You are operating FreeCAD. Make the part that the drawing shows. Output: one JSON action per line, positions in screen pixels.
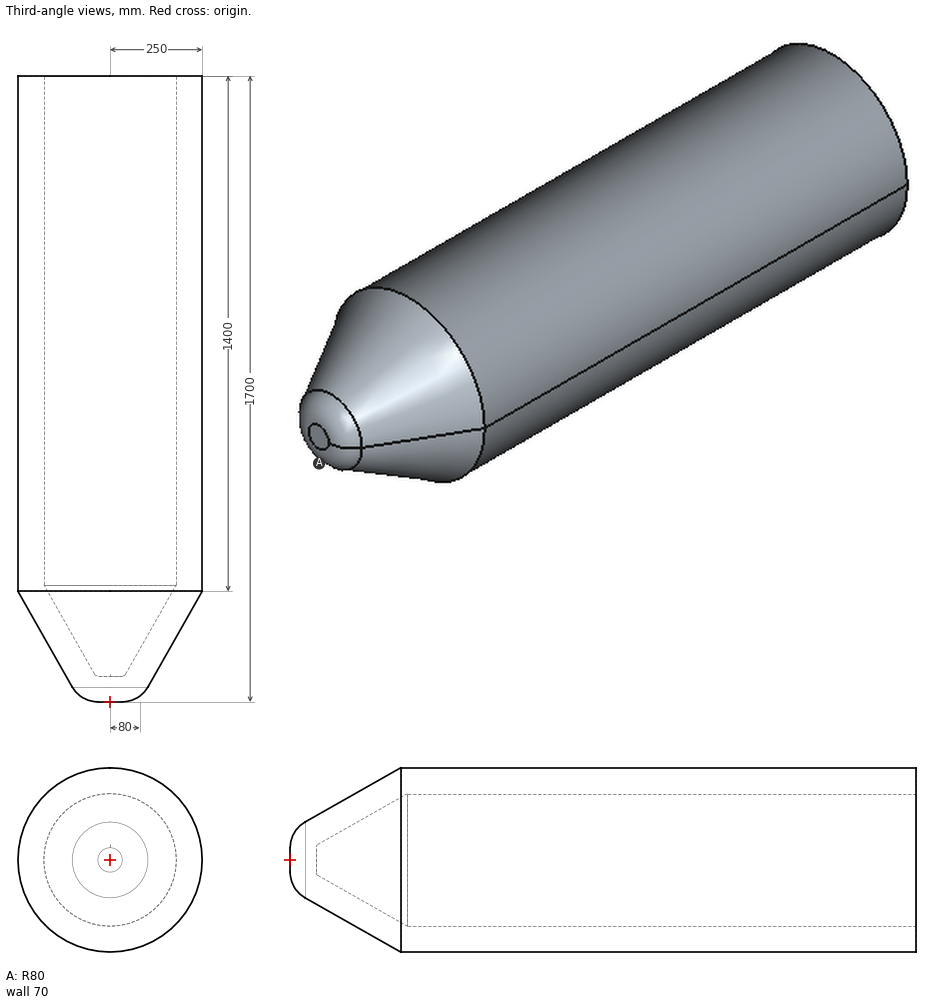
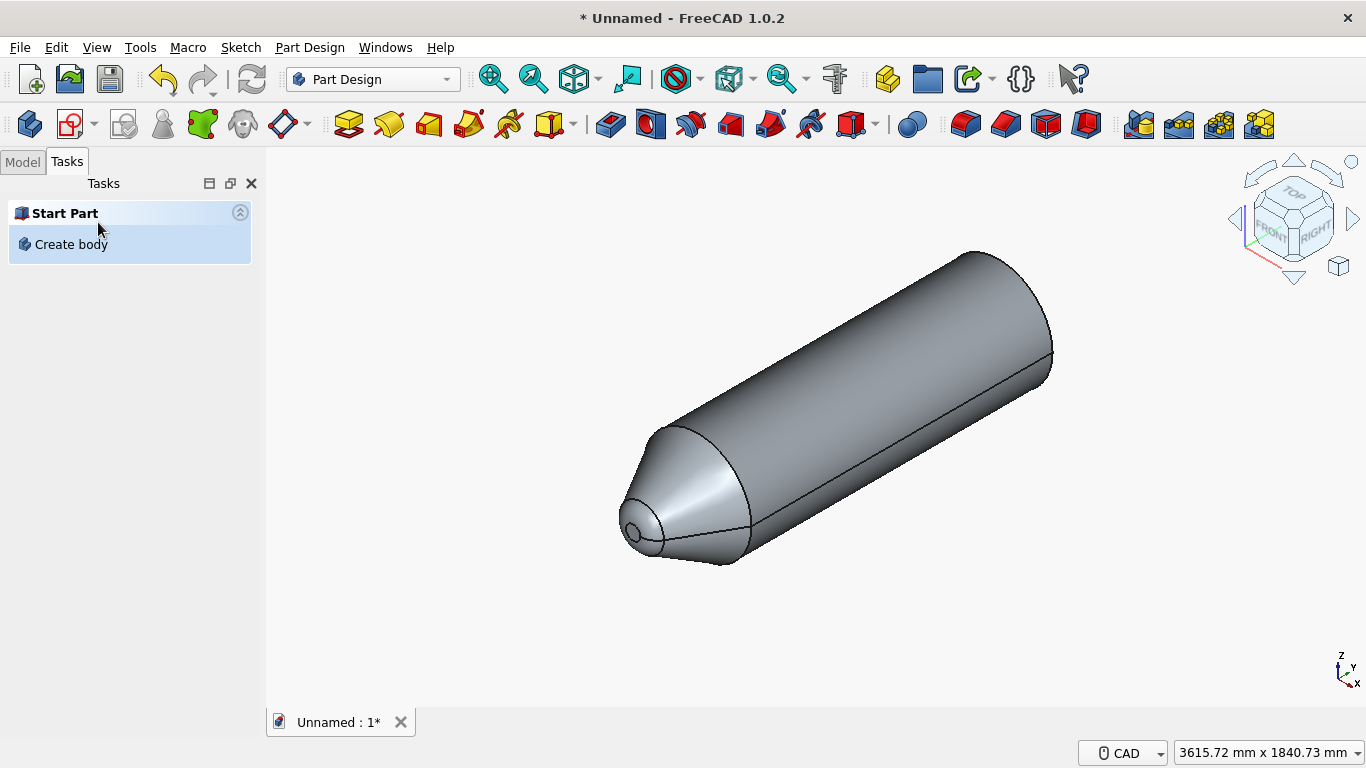
{"action": "key", "text": "2"}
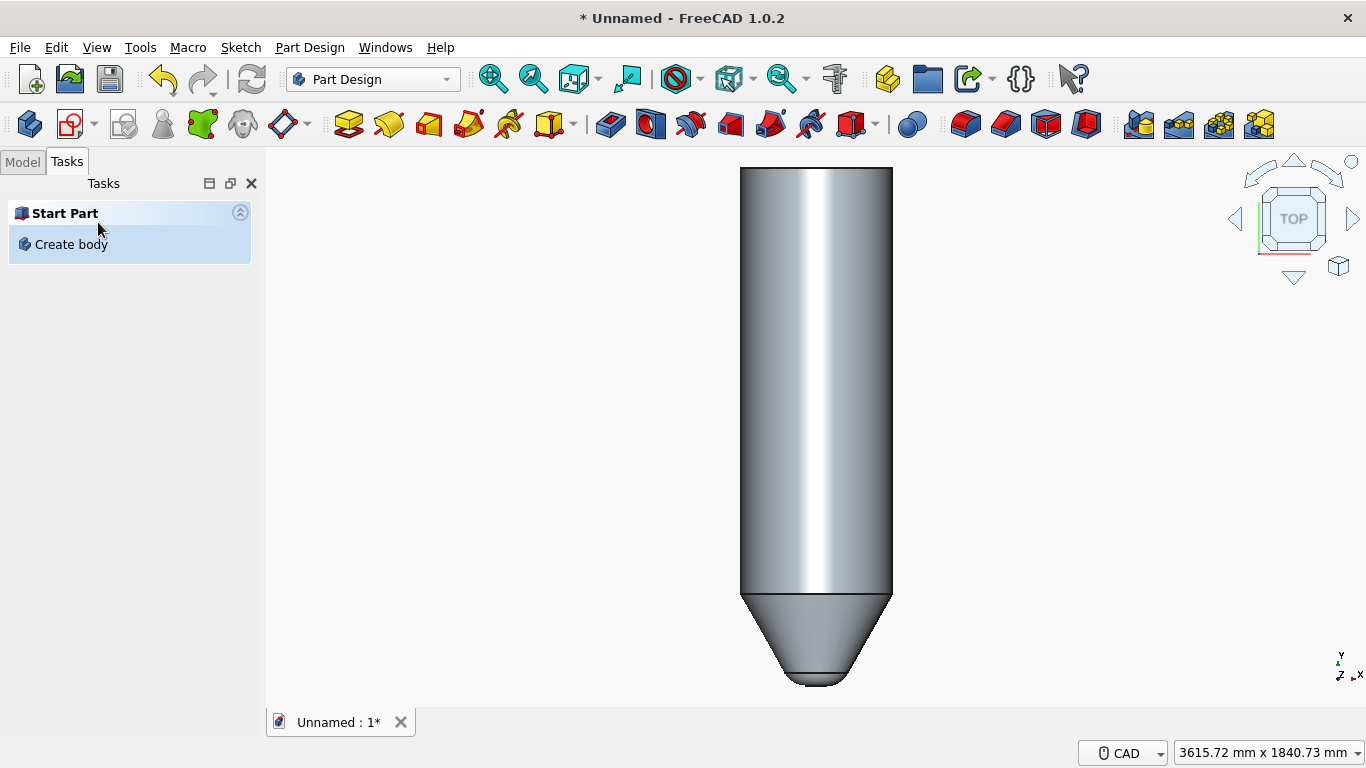
{"action": "key", "text": "1"}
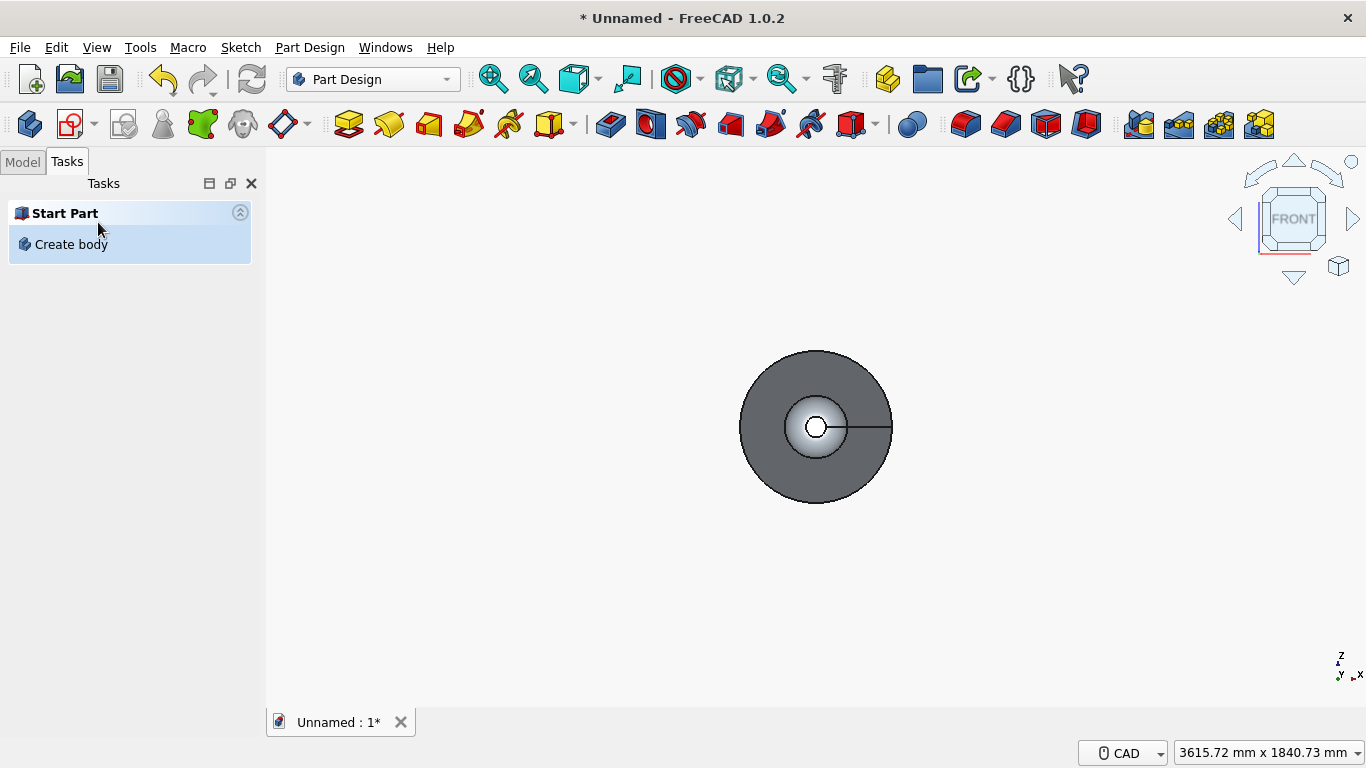
{"action": "left_click", "coordinate": [494, 80]}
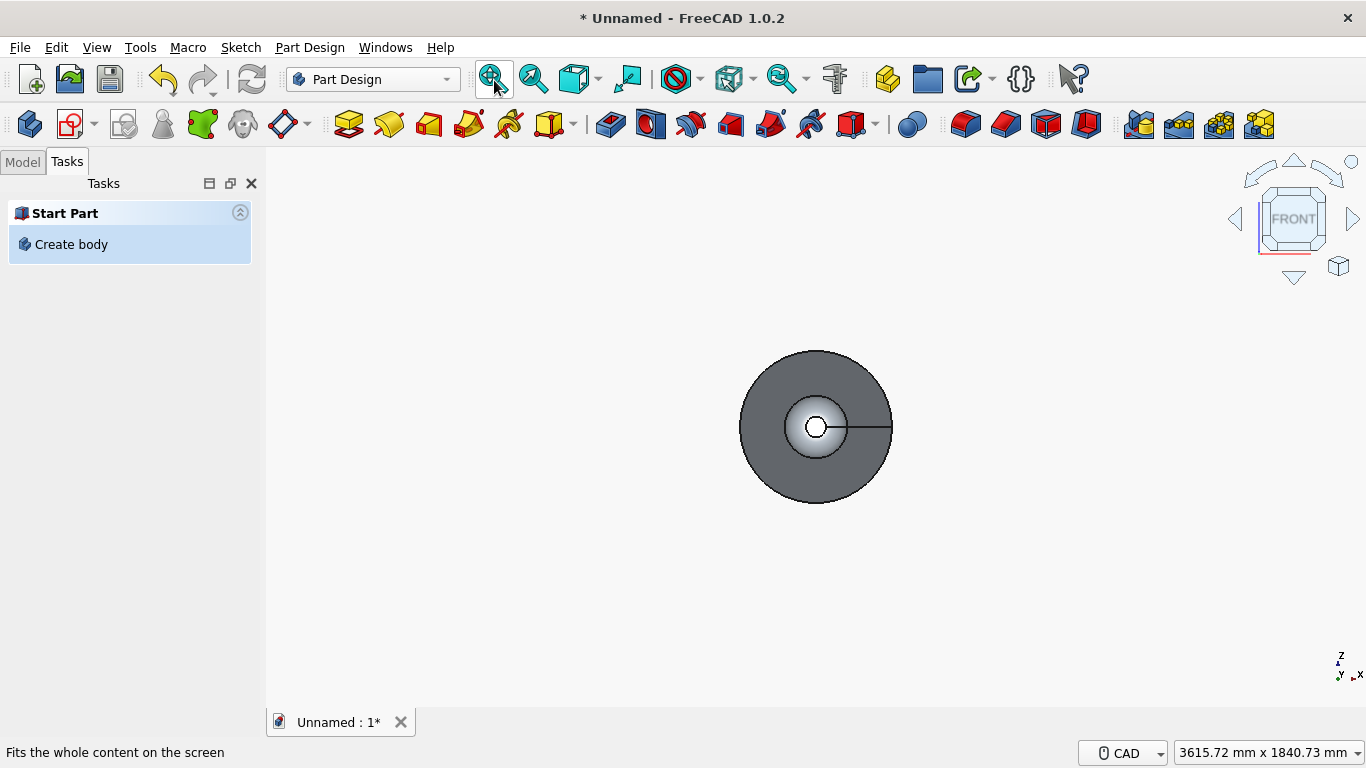
{"action": "key", "text": "3"}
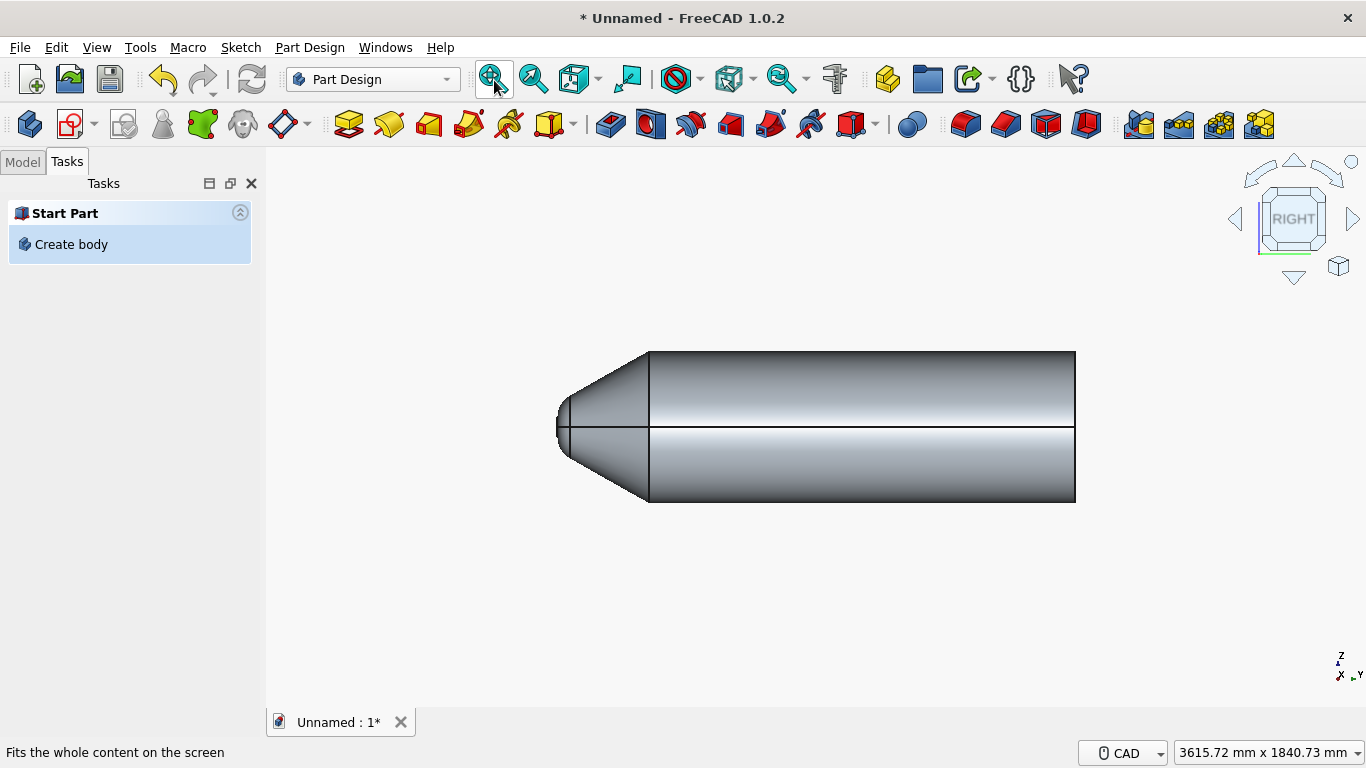
{"action": "key", "text": "5"}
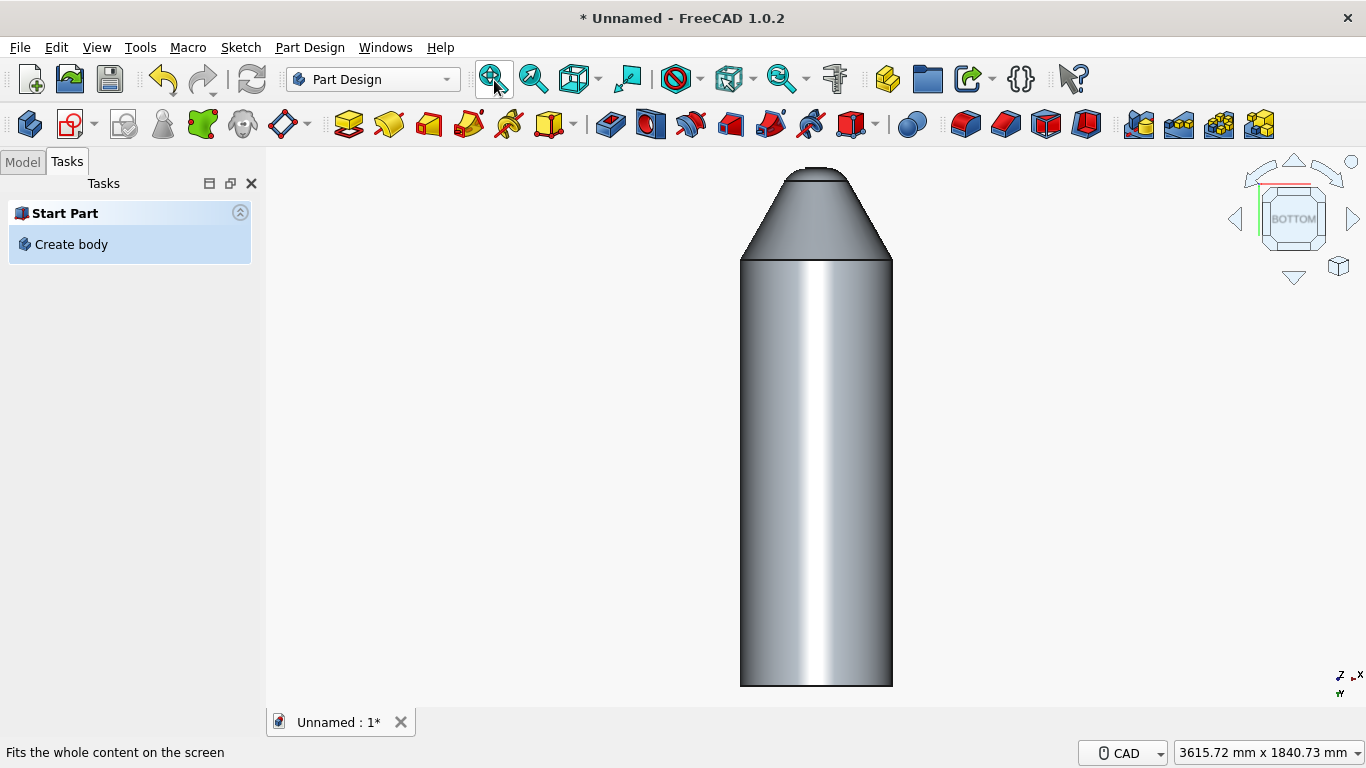
{"action": "key", "text": "4"}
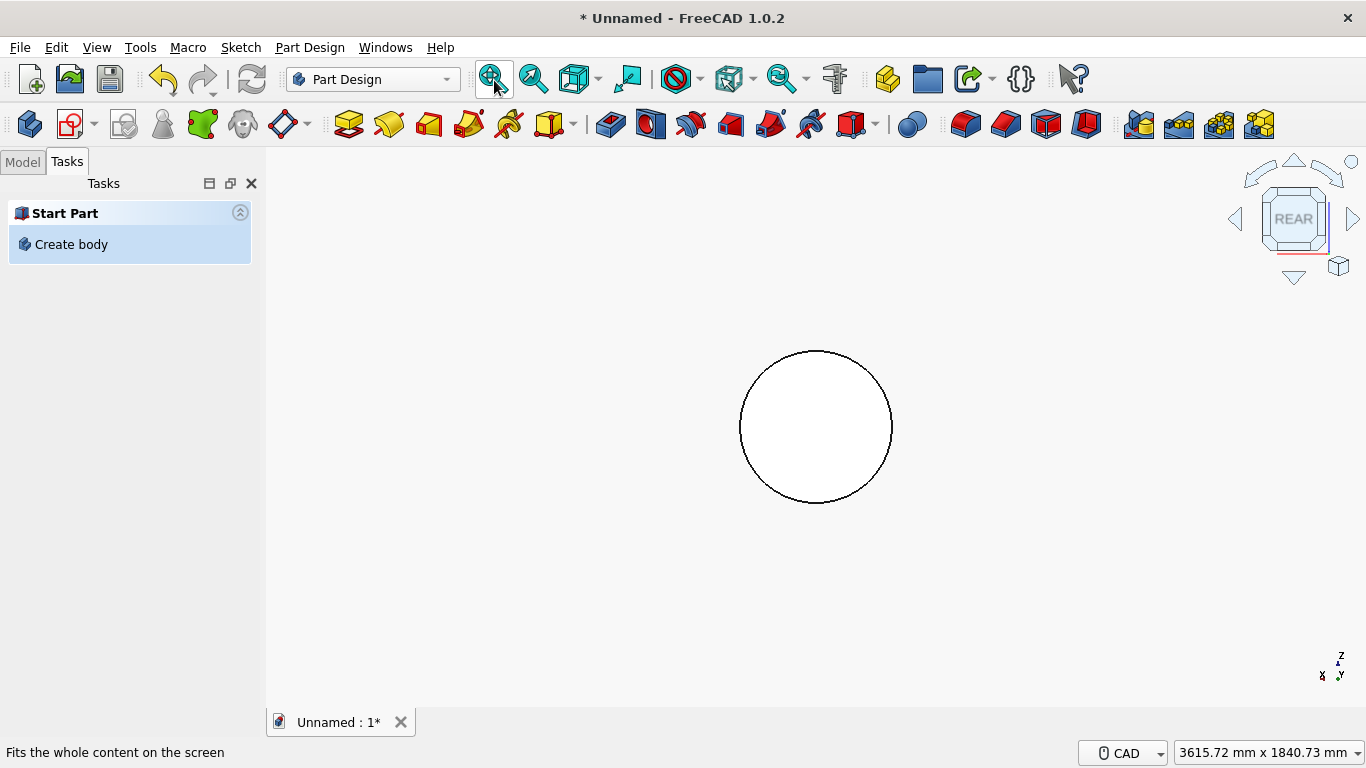
{"action": "key", "text": "v f"}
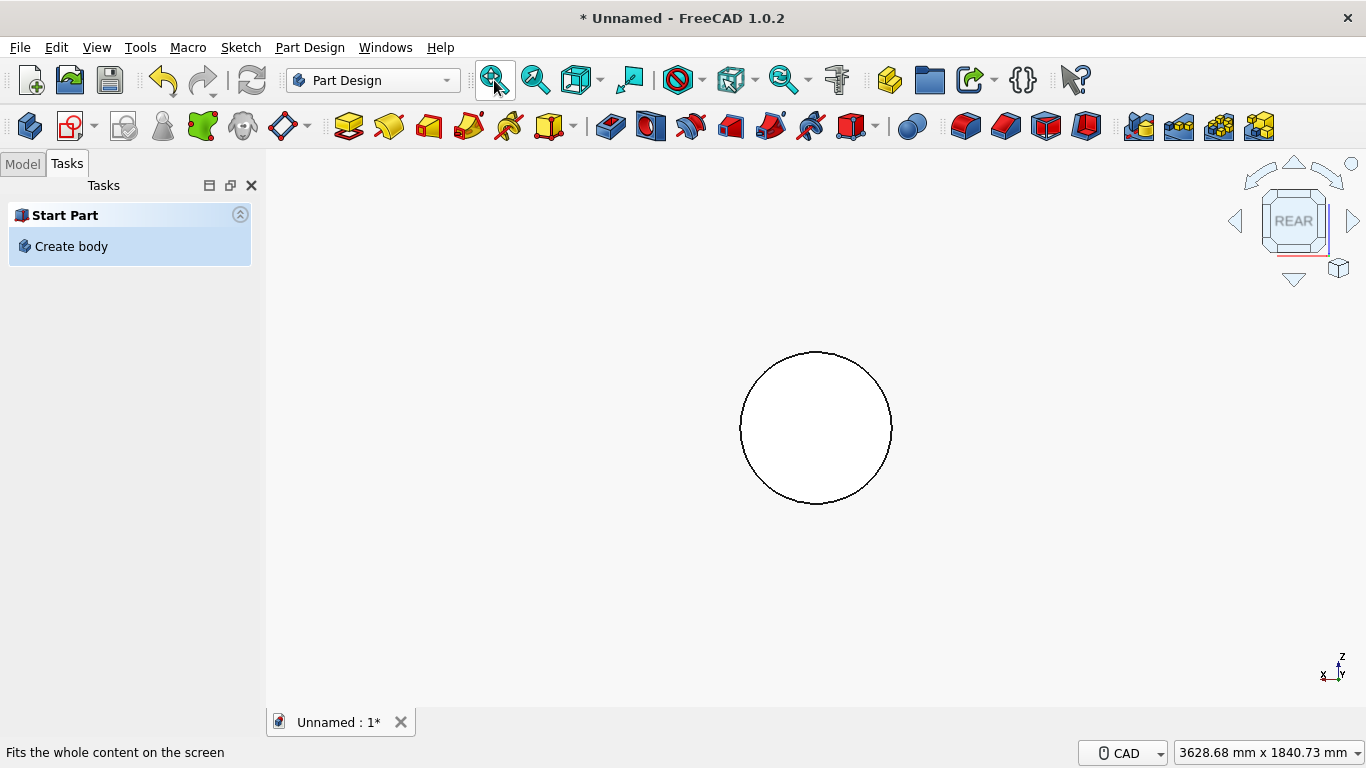
{"action": "left_click", "coordinate": [816, 427]}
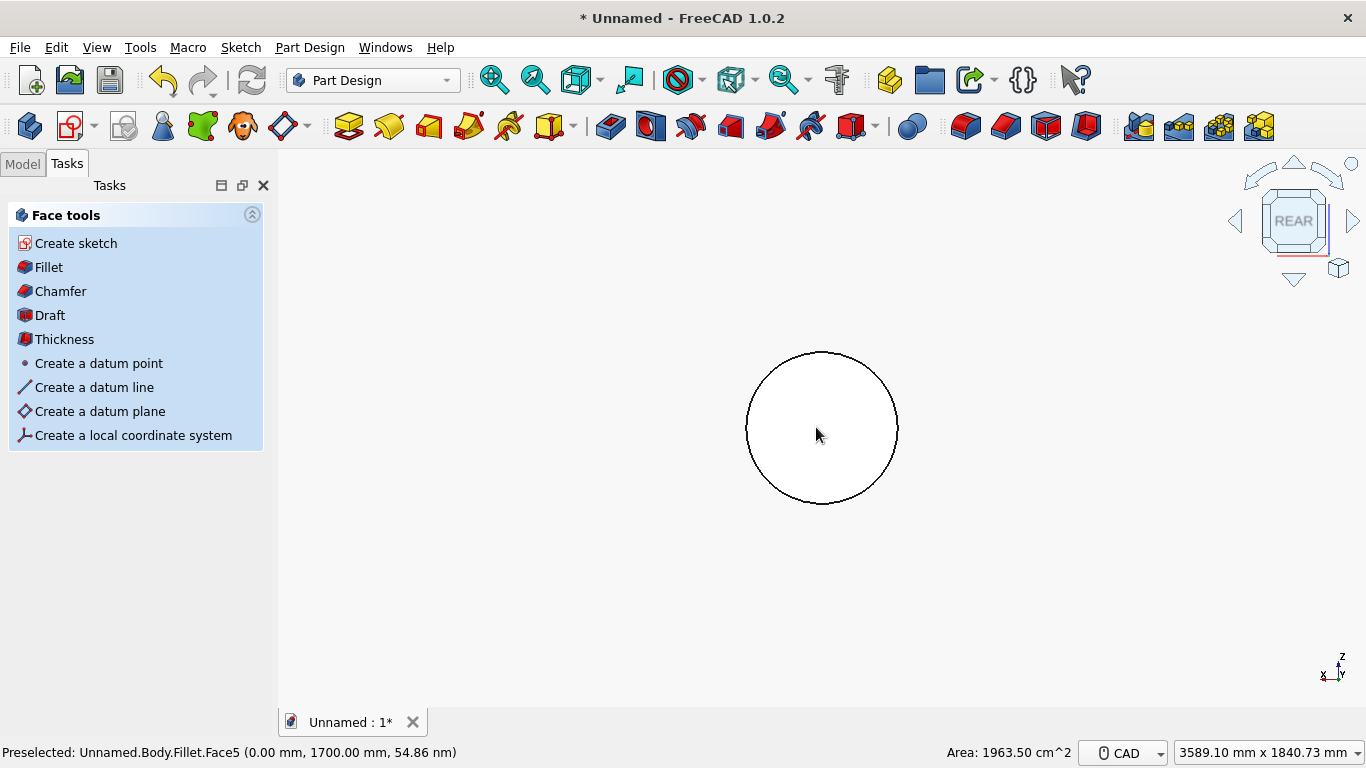
{"action": "left_click", "coordinate": [1086, 126]}